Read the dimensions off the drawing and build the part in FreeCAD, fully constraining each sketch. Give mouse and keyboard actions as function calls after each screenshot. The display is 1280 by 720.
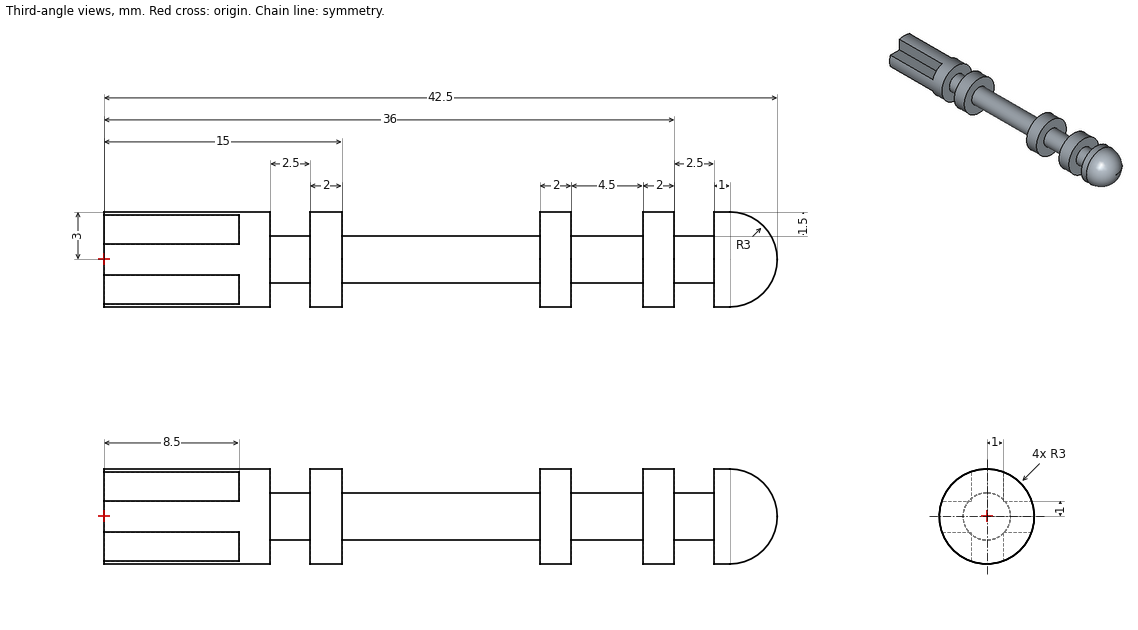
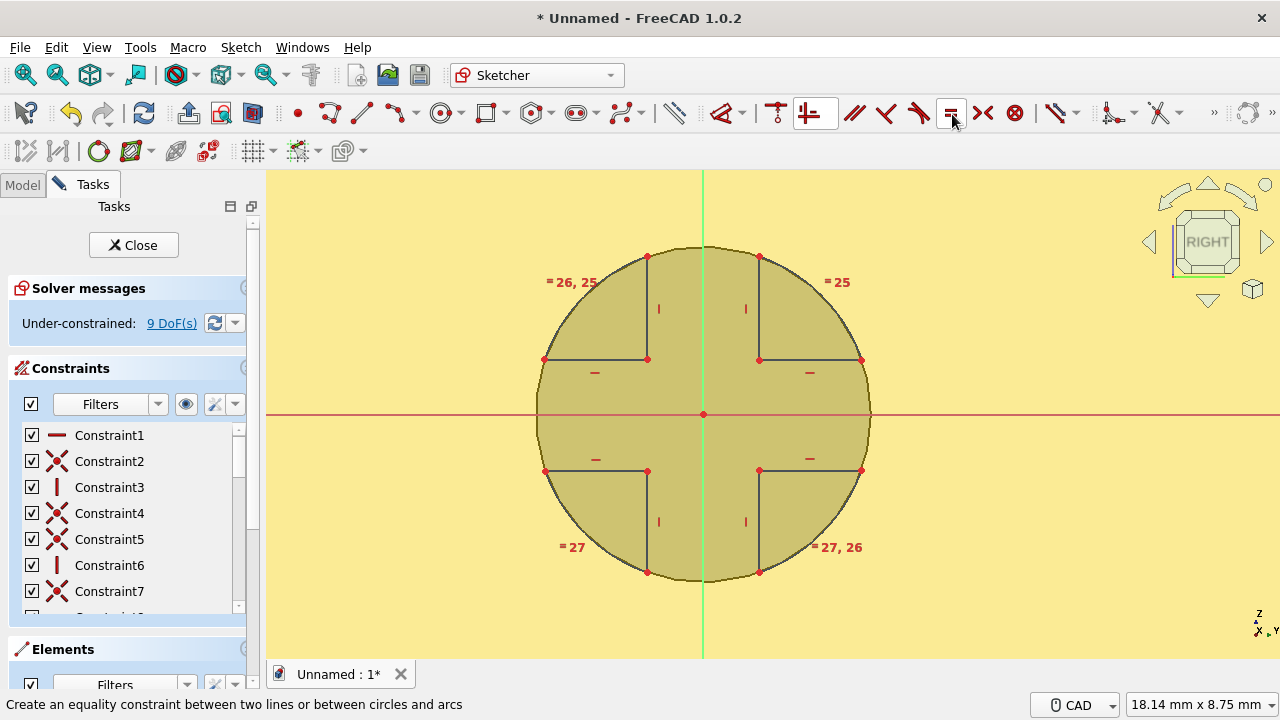
click(759, 360)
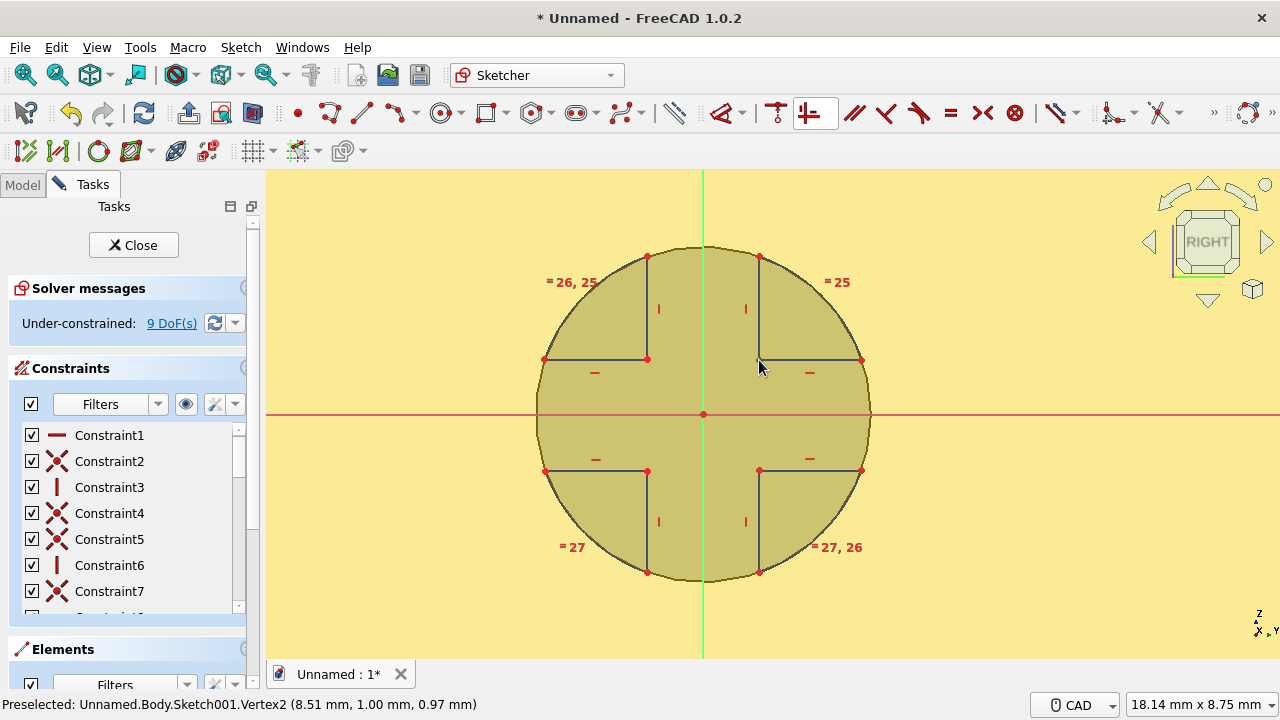
click(647, 360)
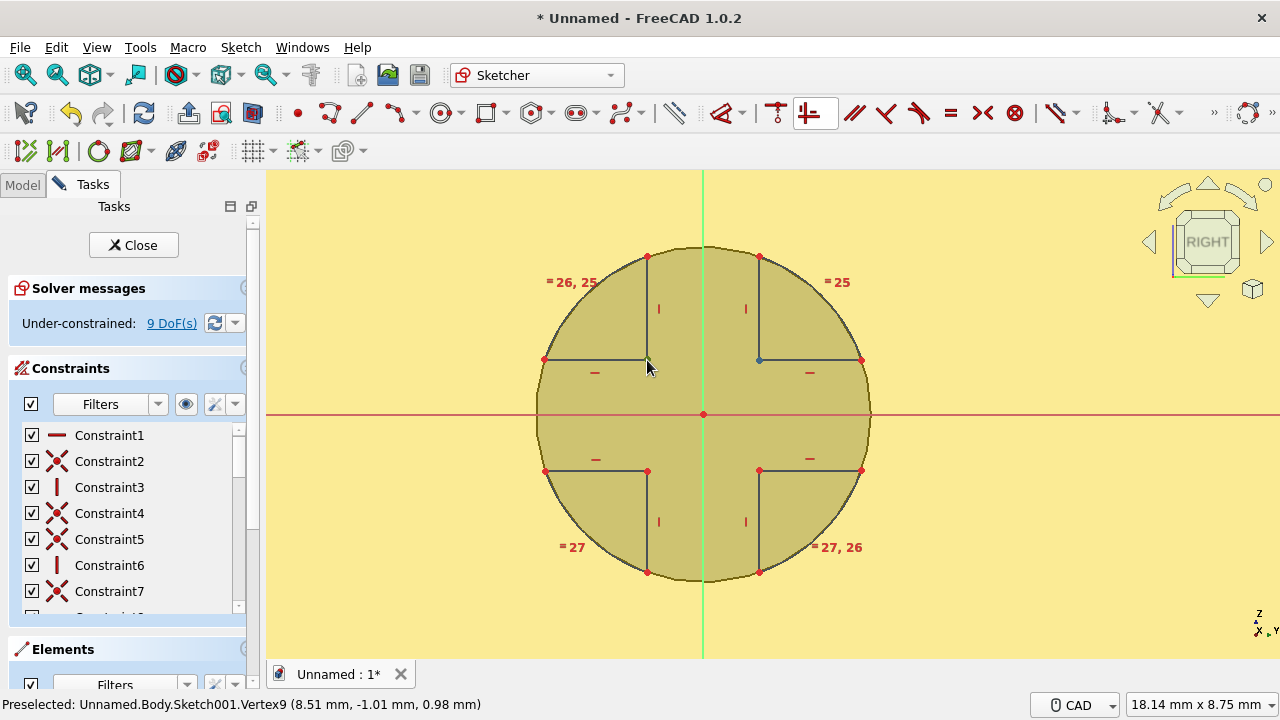
click(703, 600)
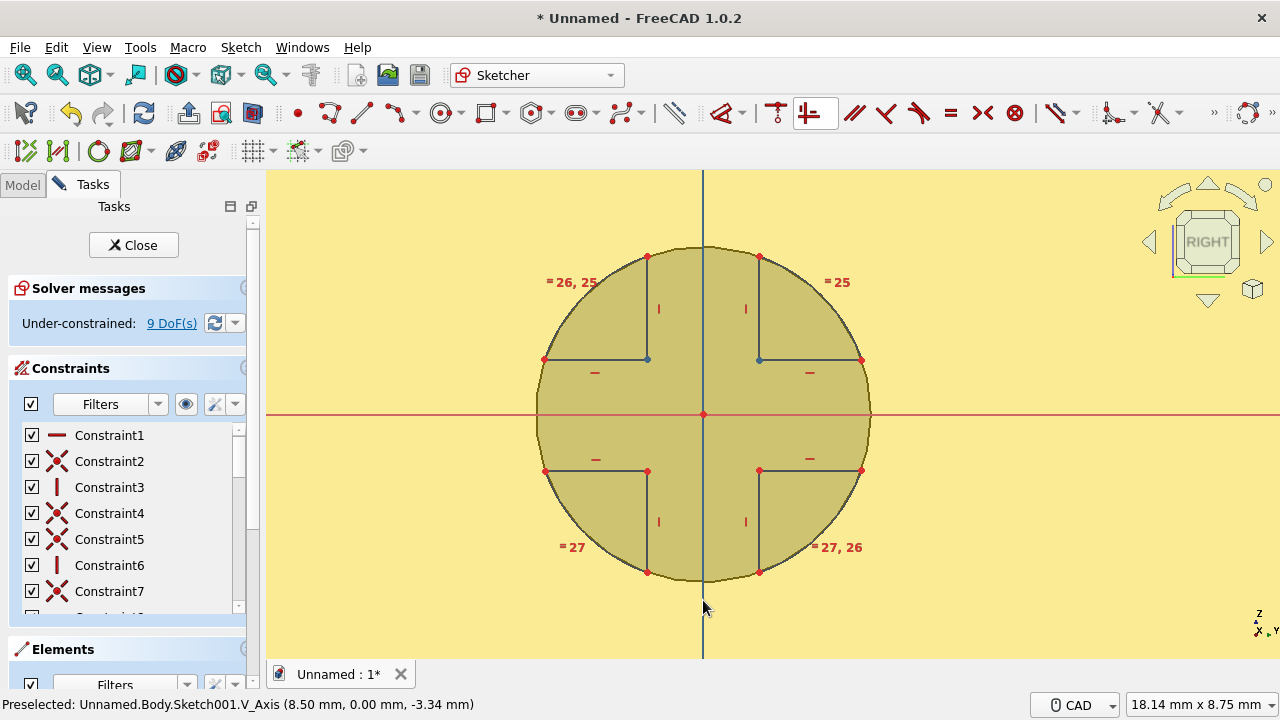
click(984, 114)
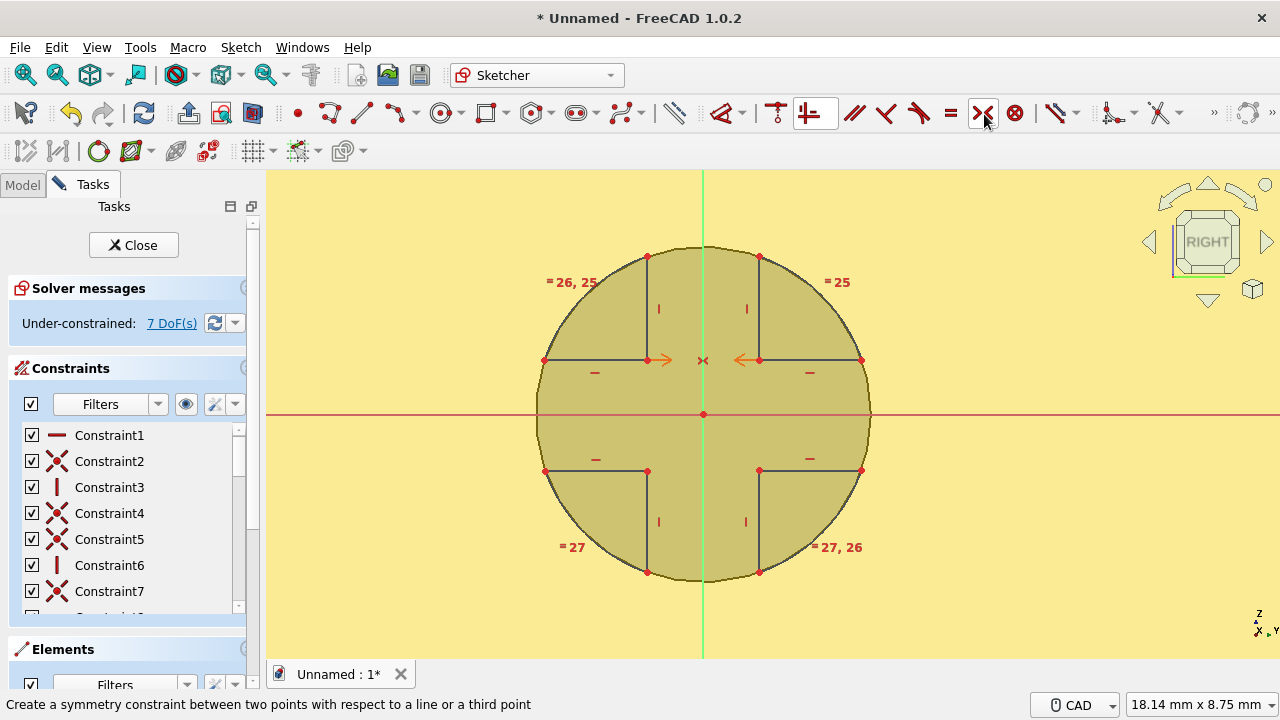
click(759, 360)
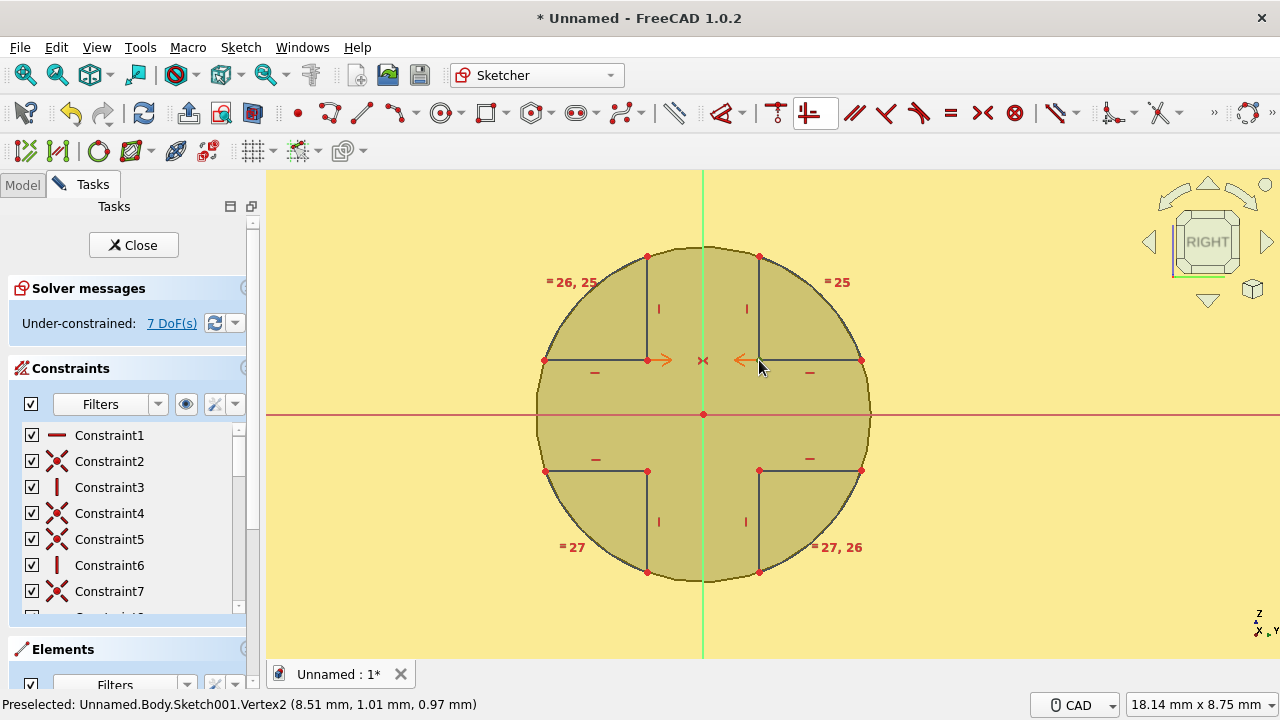
click(759, 471)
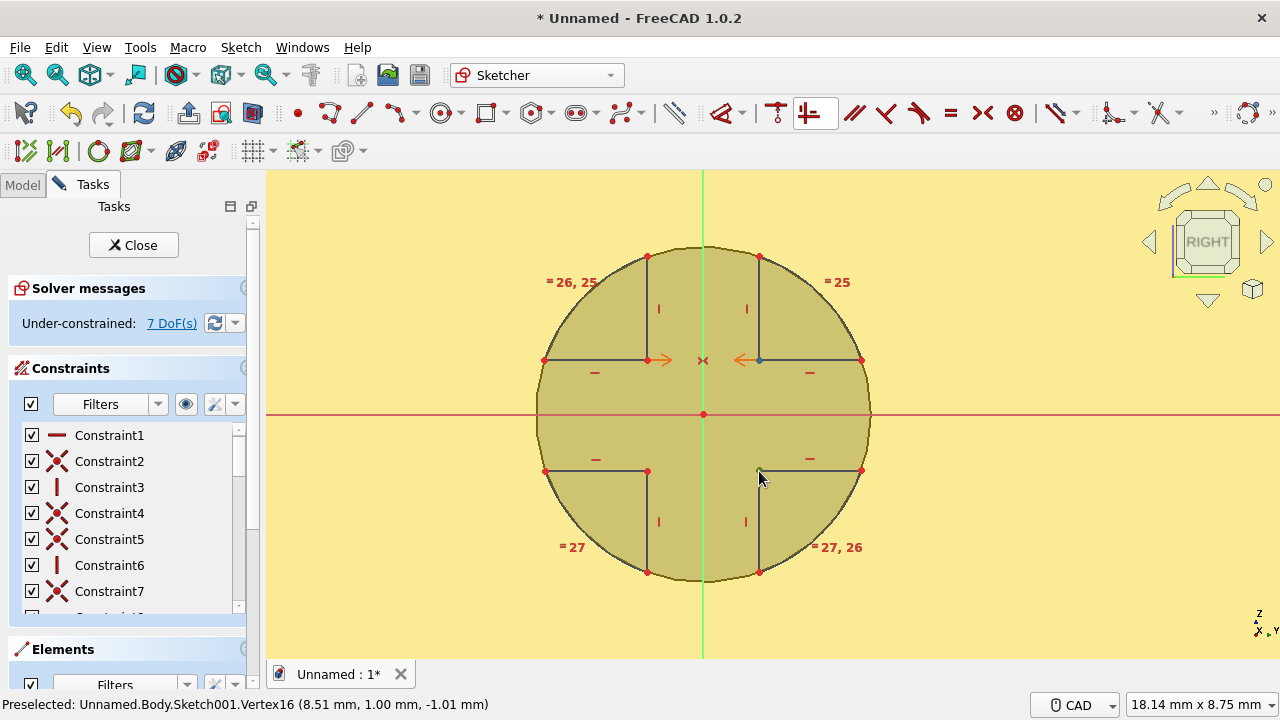
click(353, 414)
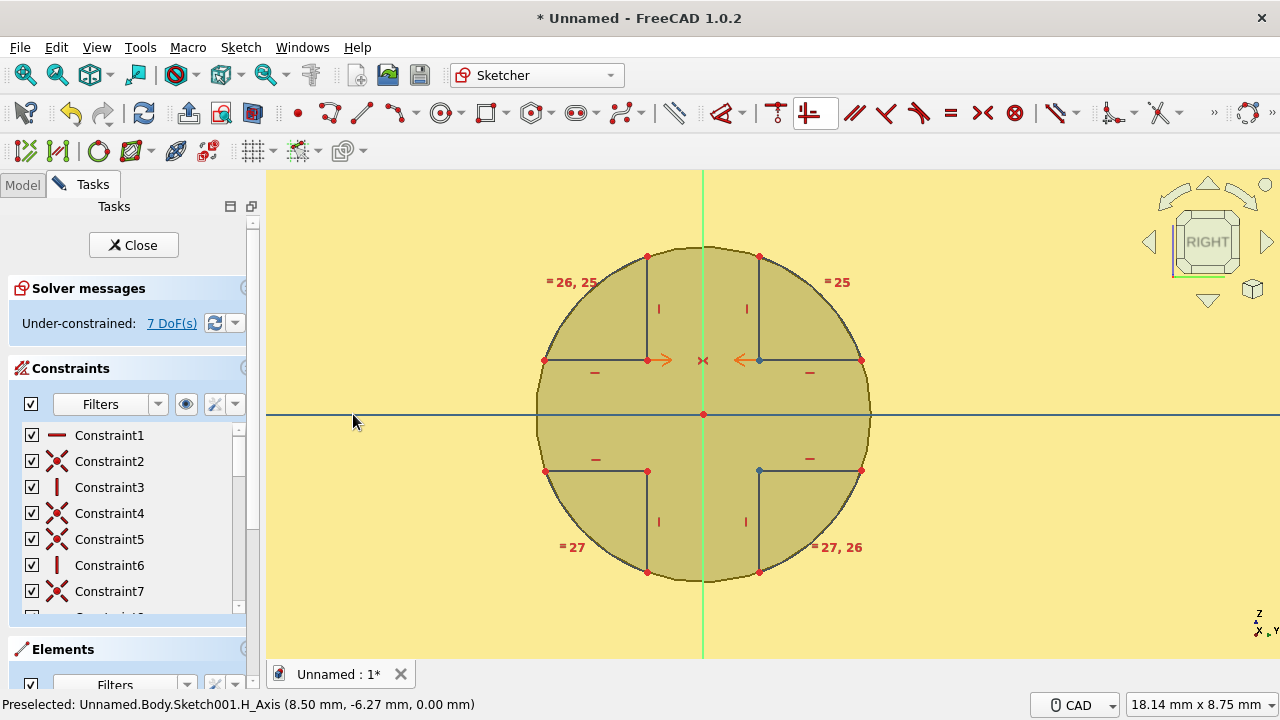
click(984, 114)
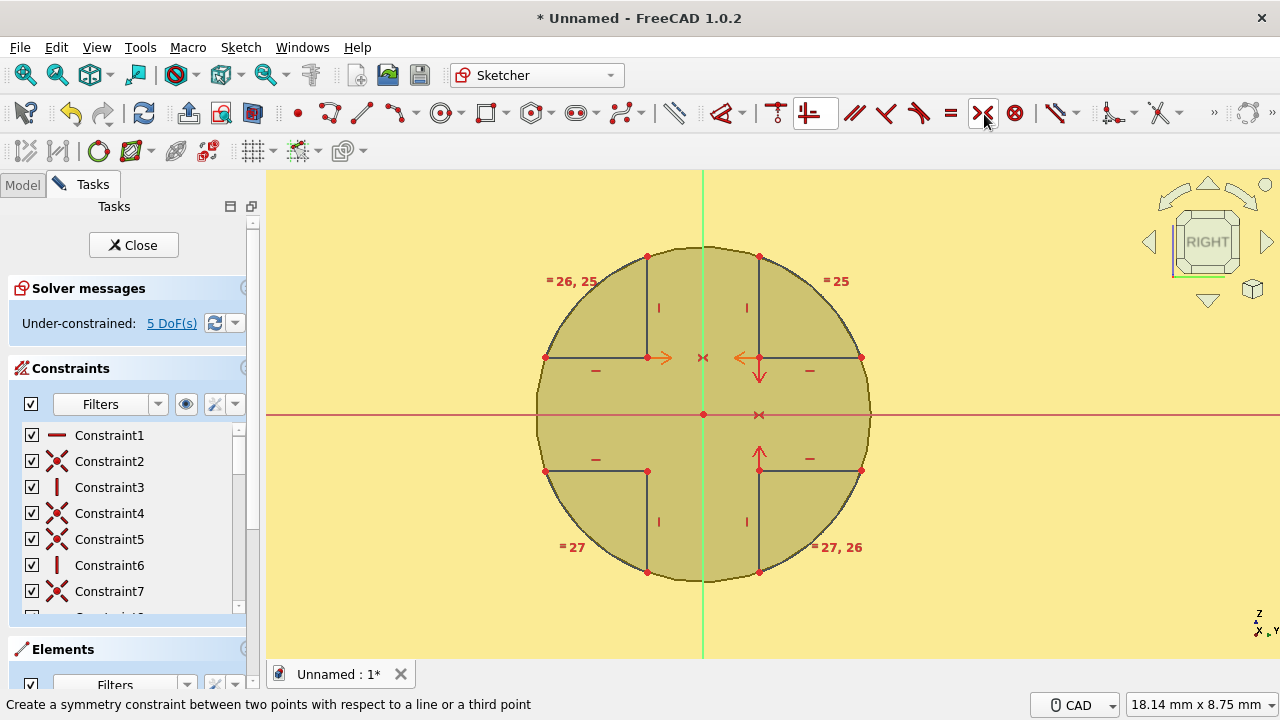
click(647, 358)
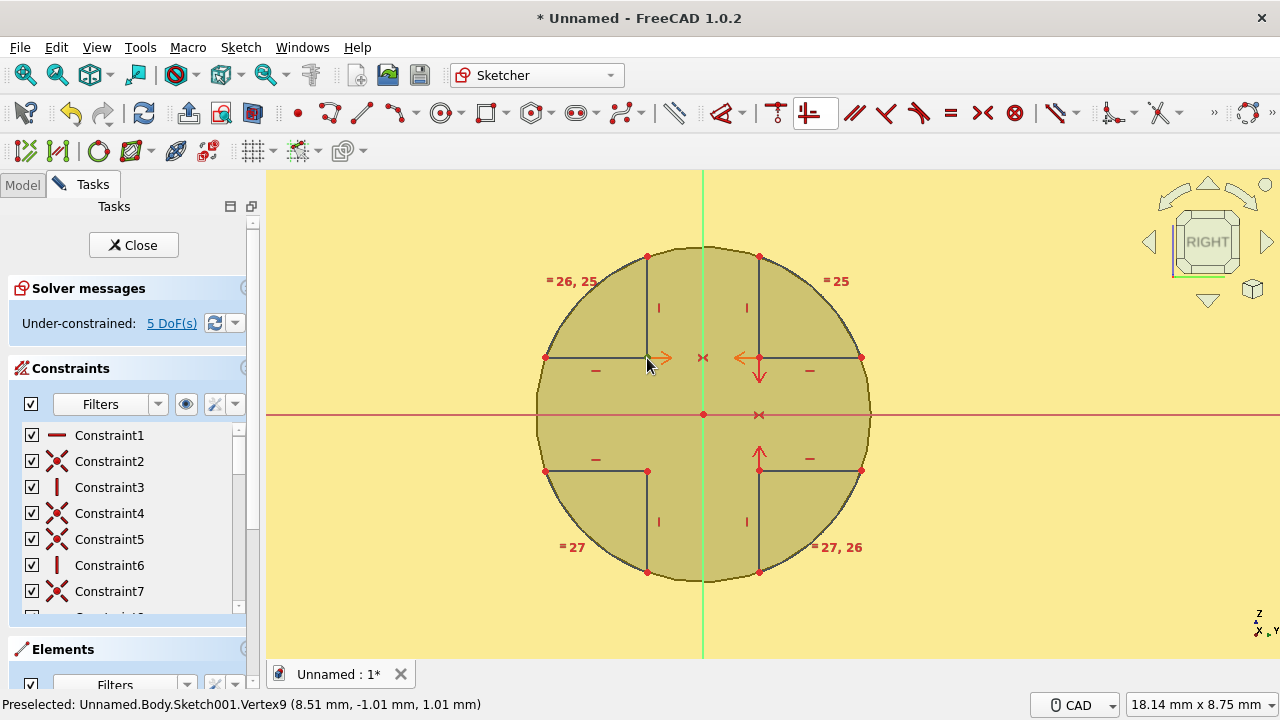
click(647, 471)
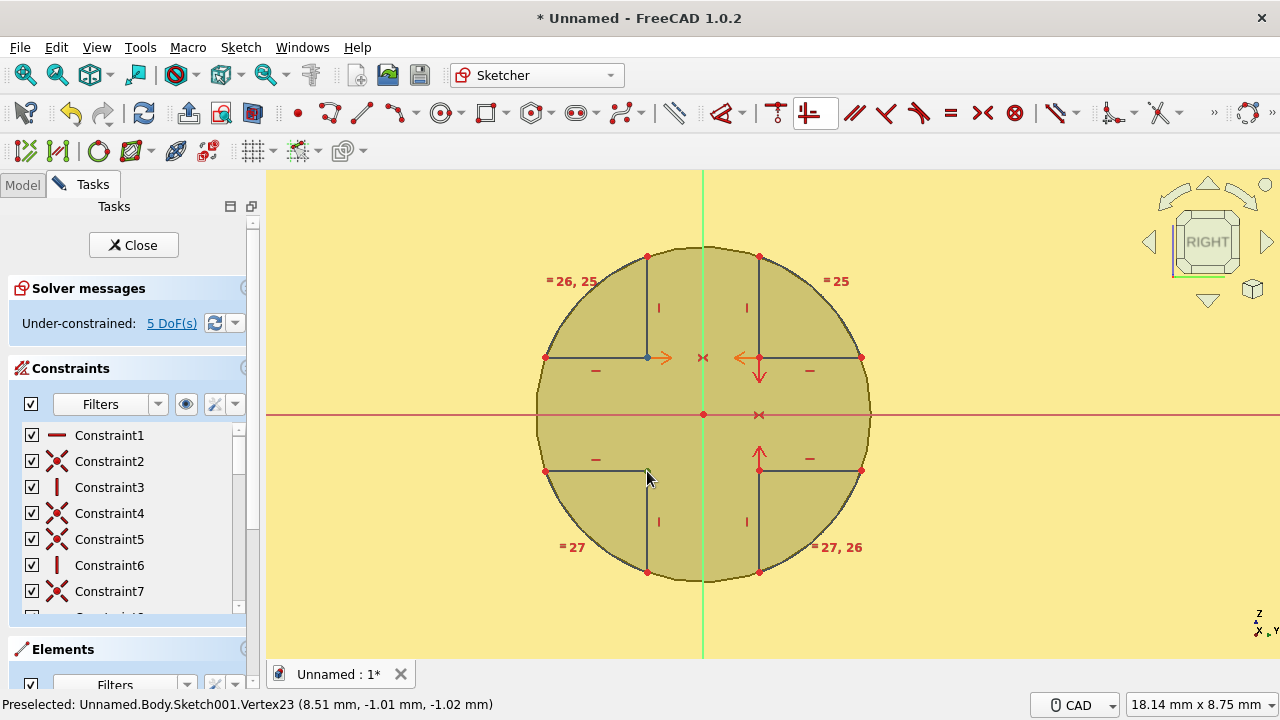
click(353, 414)